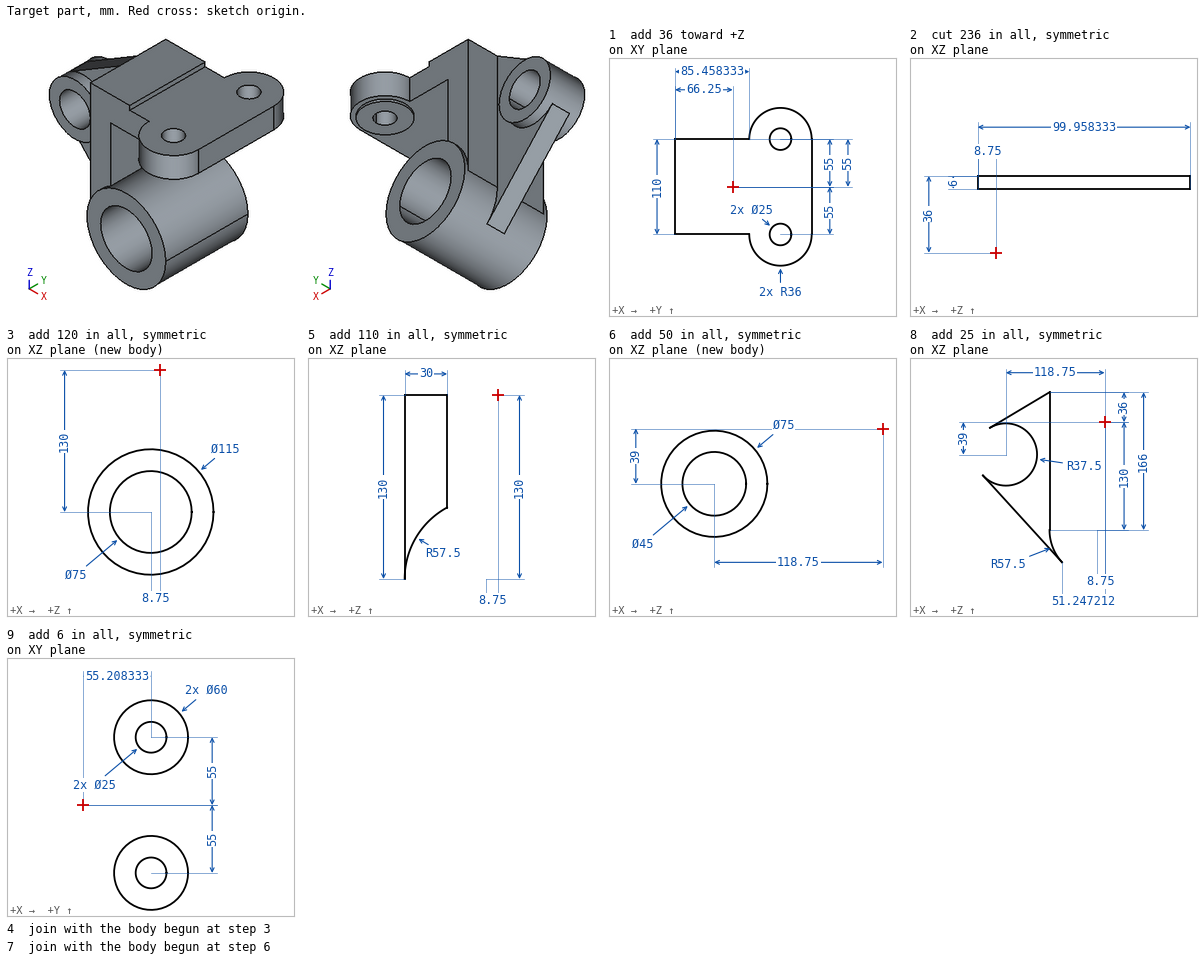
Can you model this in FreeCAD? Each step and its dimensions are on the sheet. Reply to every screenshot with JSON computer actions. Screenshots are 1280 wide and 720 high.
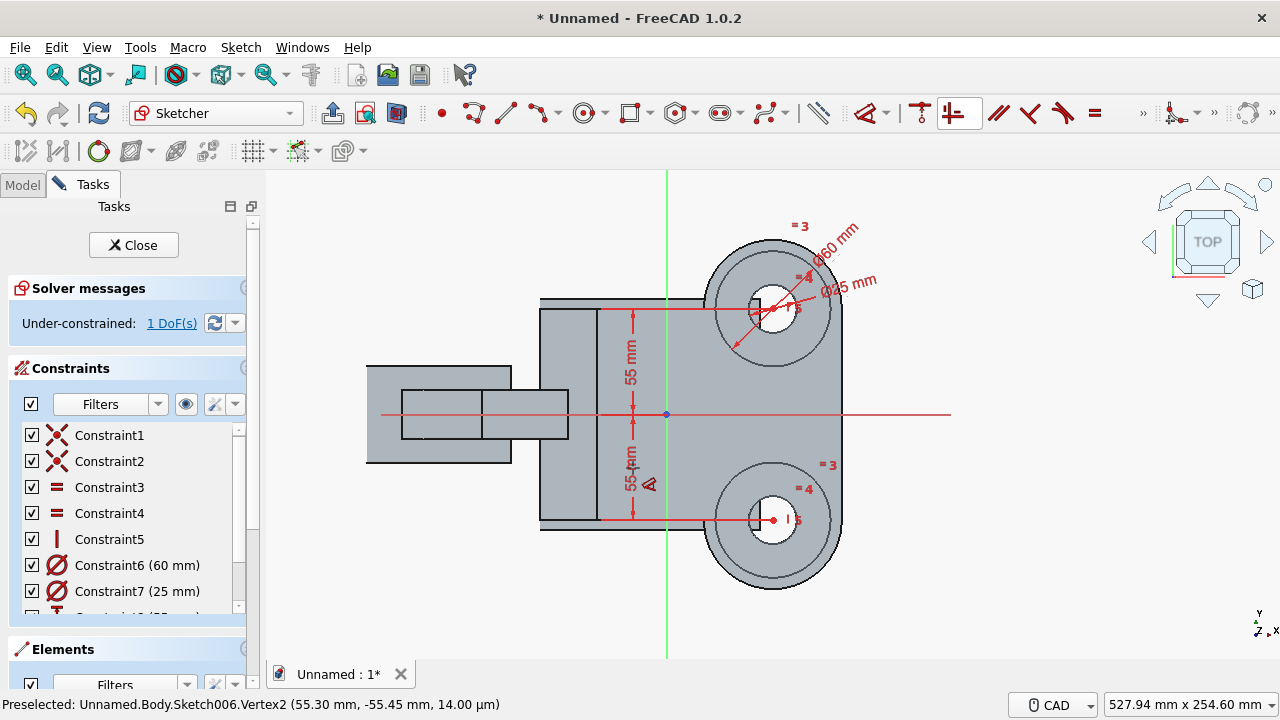
{"action": "left_click", "coordinate": [773, 309]}
{"action": "left_click", "coordinate": [695, 275]}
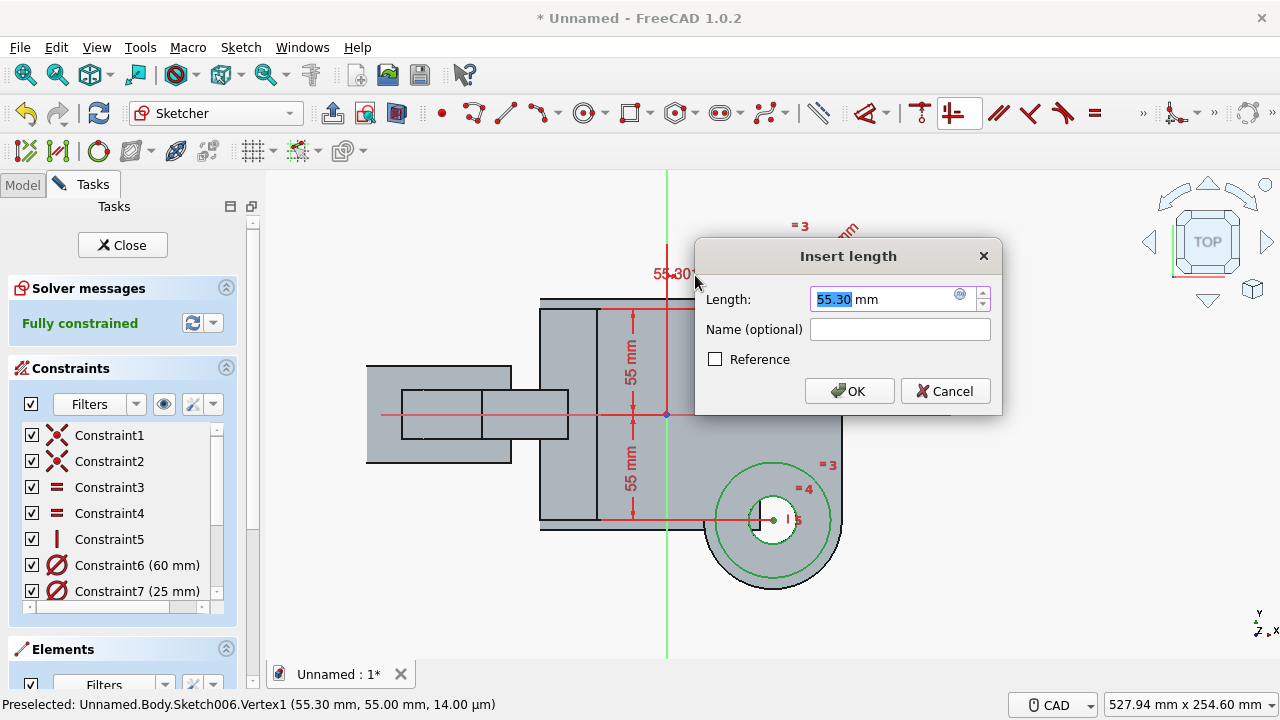
{"action": "type", "text": "55.208333"}
{"action": "key", "text": "Return"}
{"action": "key", "text": "Escape"}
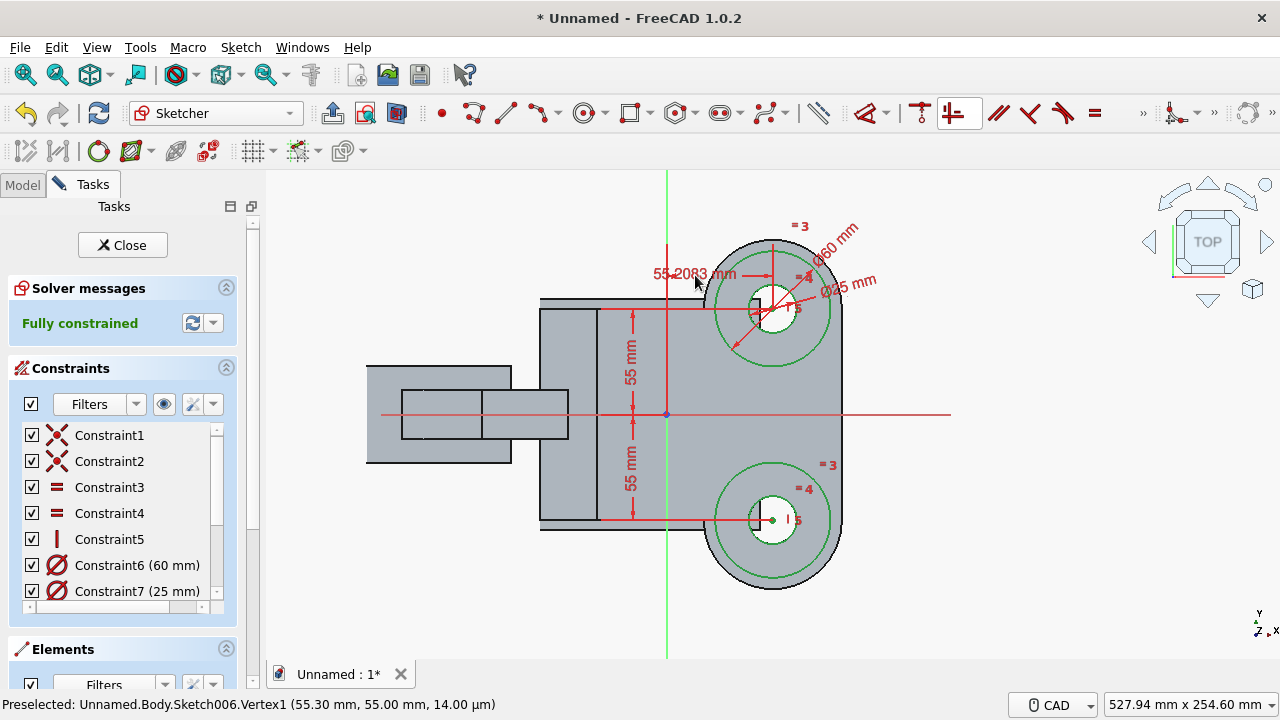
{"action": "left_click", "coordinate": [123, 245]}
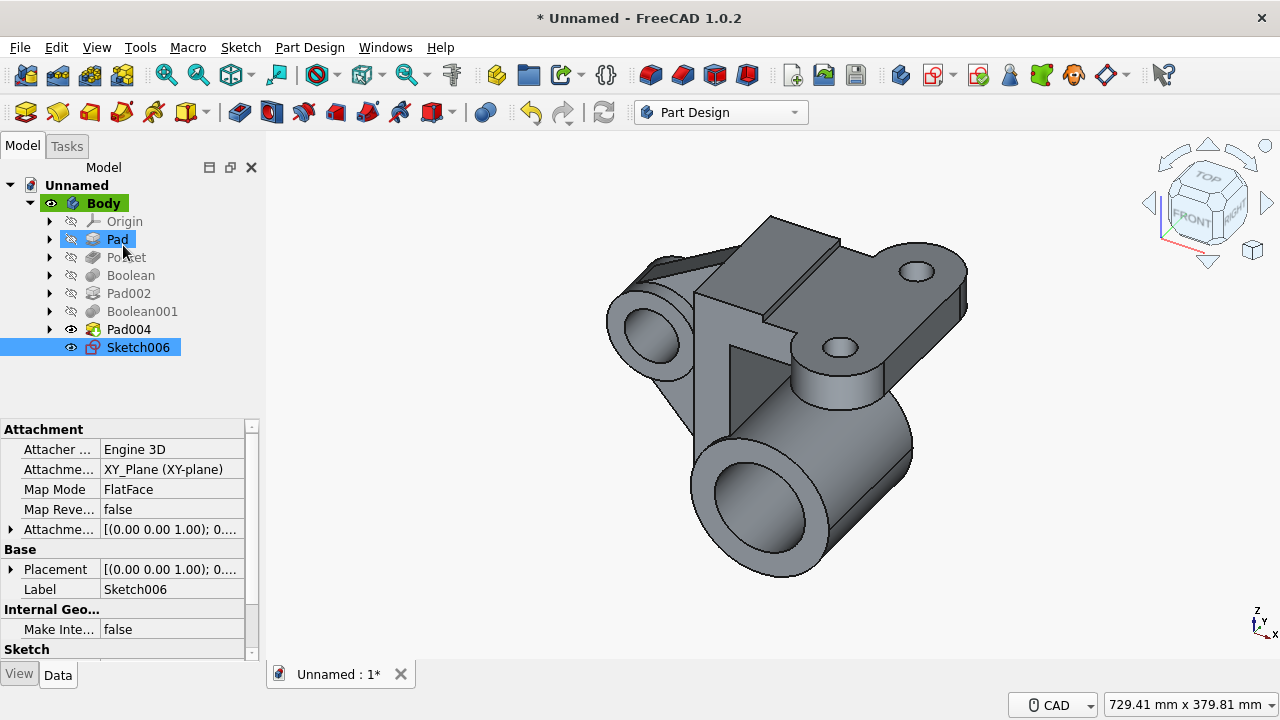
{"action": "left_click", "coordinate": [26, 112]}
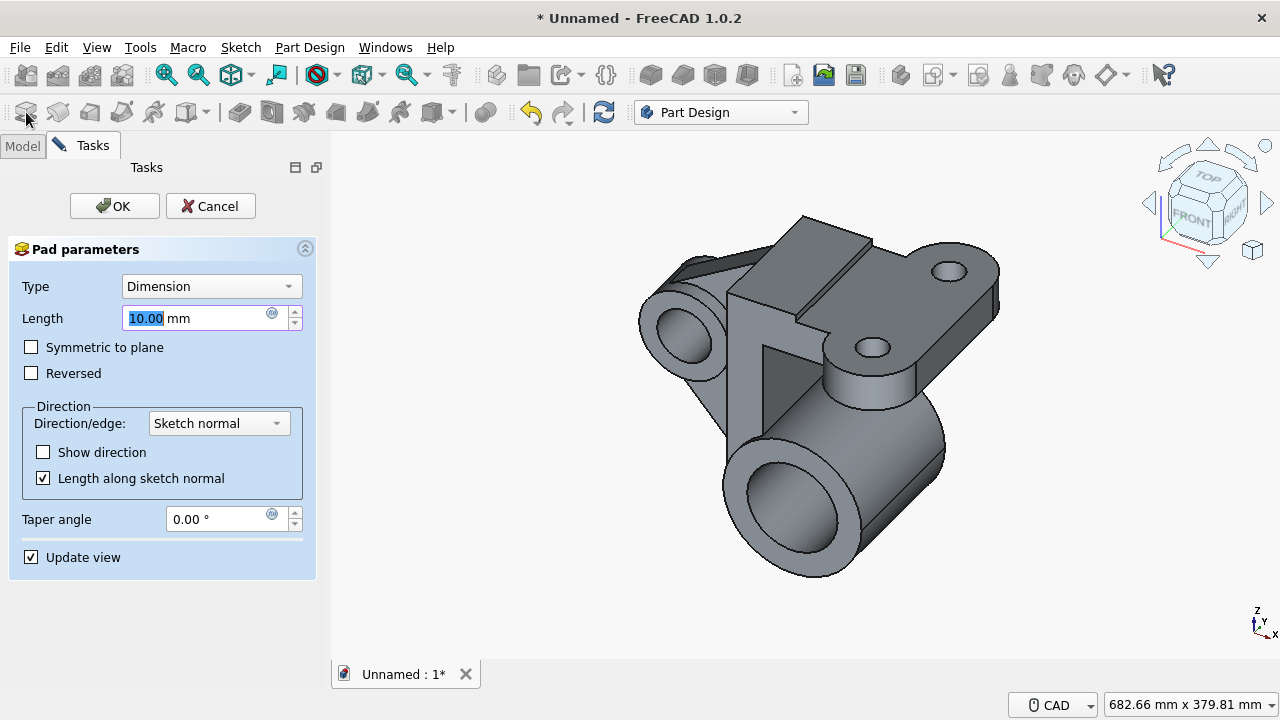
{"action": "type", "text": "6"}
{"action": "key", "text": "Tab"}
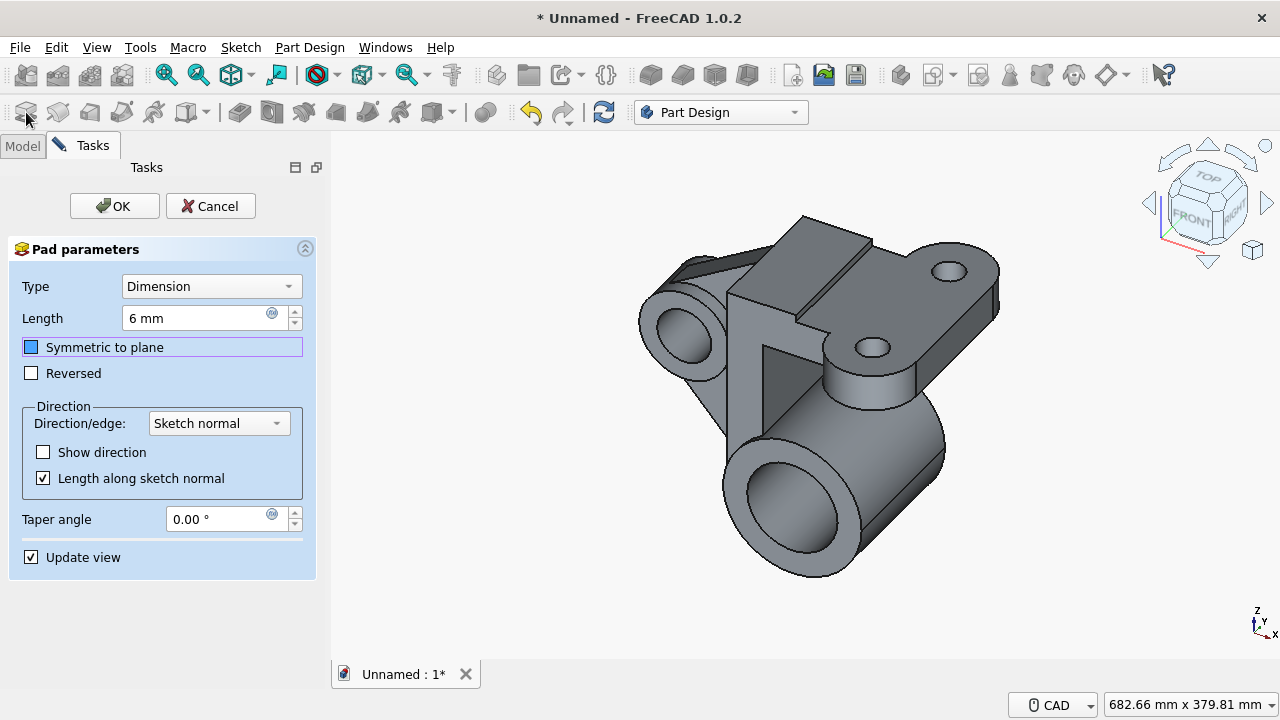
{"action": "left_click", "coordinate": [30, 347]}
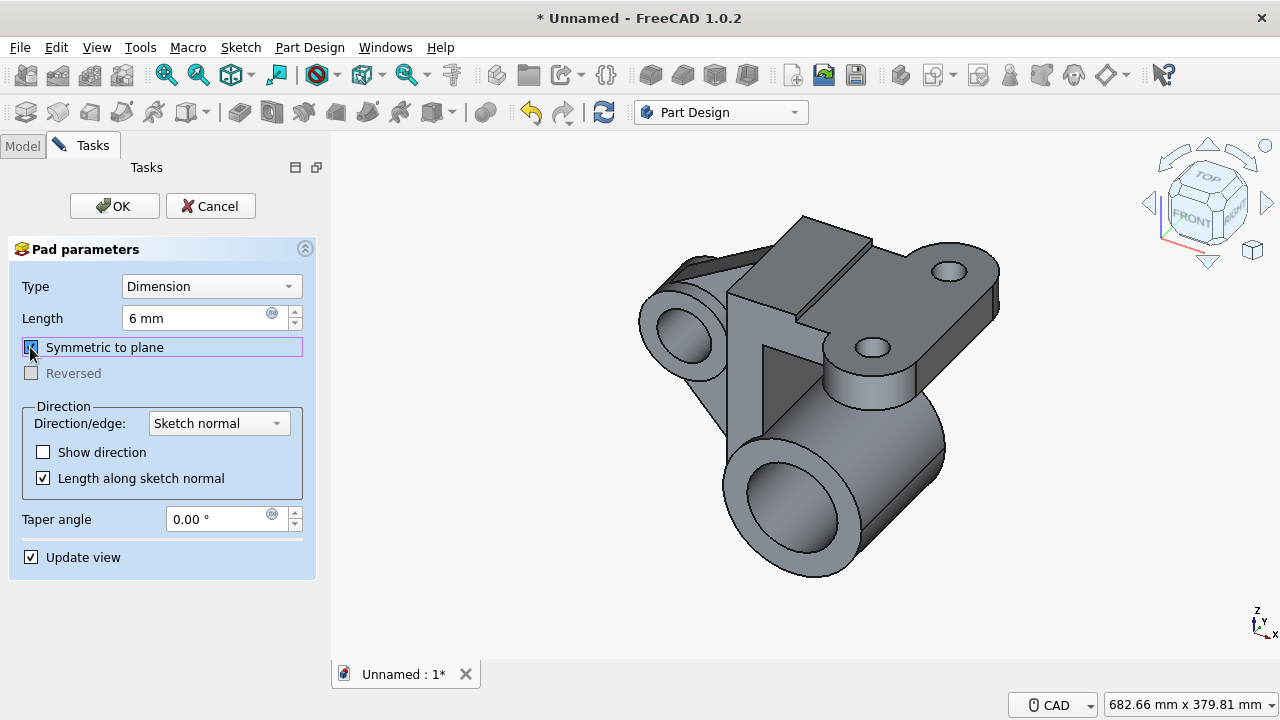
{"action": "left_click", "coordinate": [115, 206]}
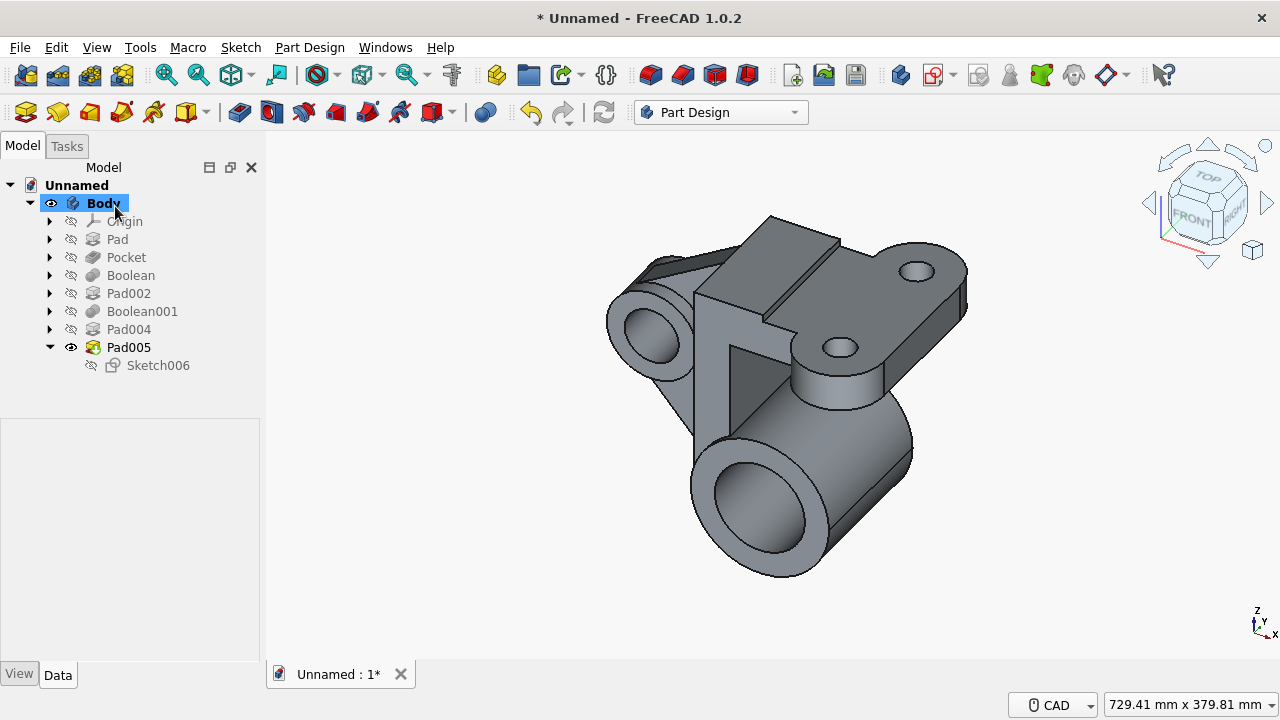
{"action": "key", "text": "0"}